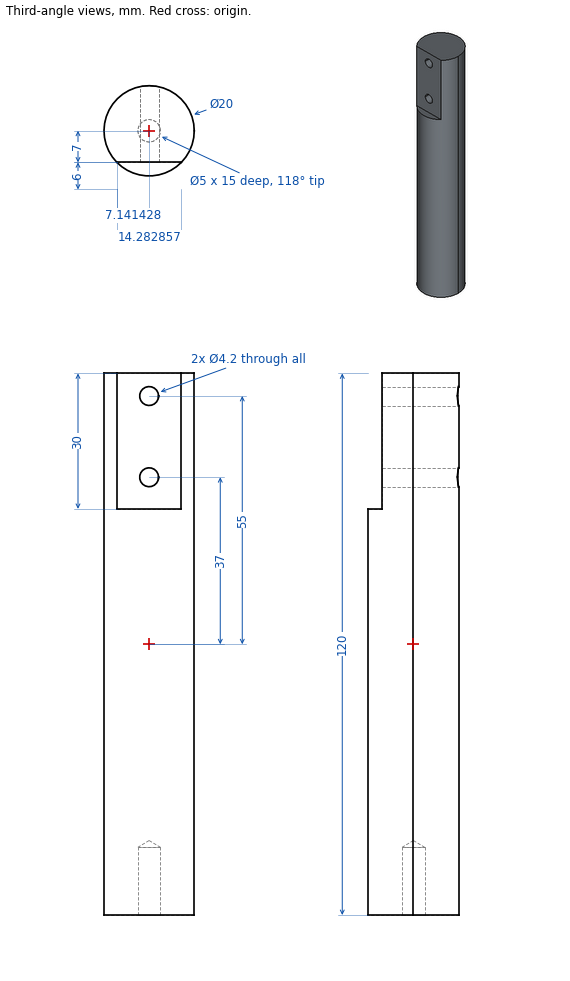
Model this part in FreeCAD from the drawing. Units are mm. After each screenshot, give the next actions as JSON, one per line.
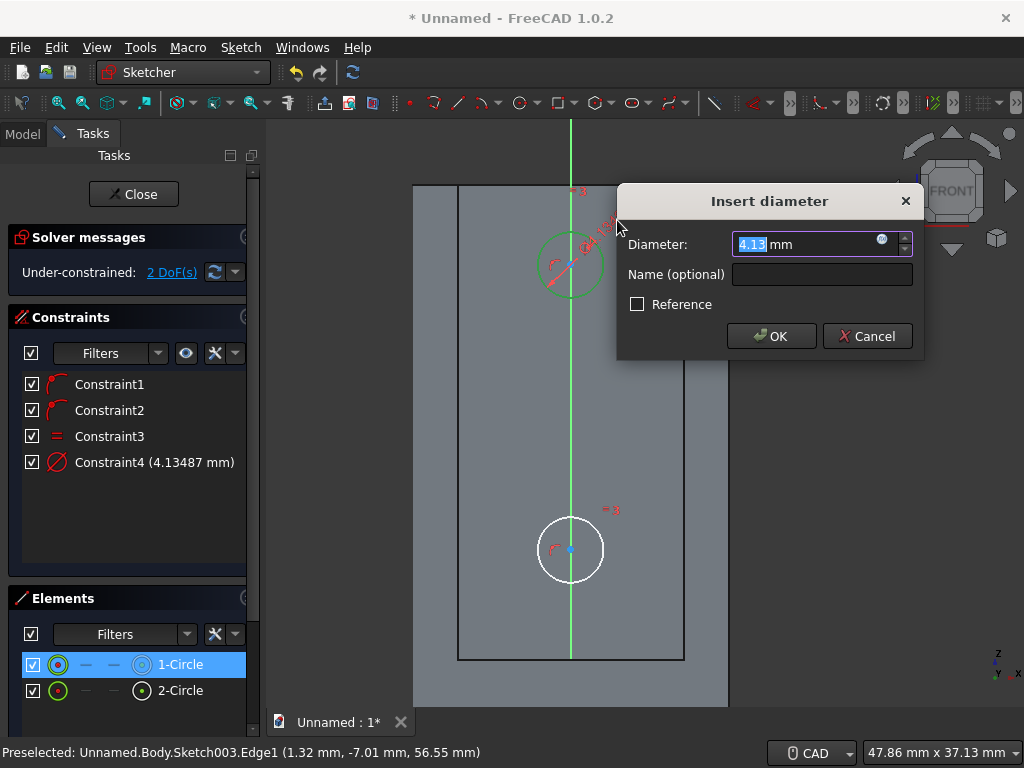
{"action": "type", "text": "4.2"}
{"action": "key", "text": "Return"}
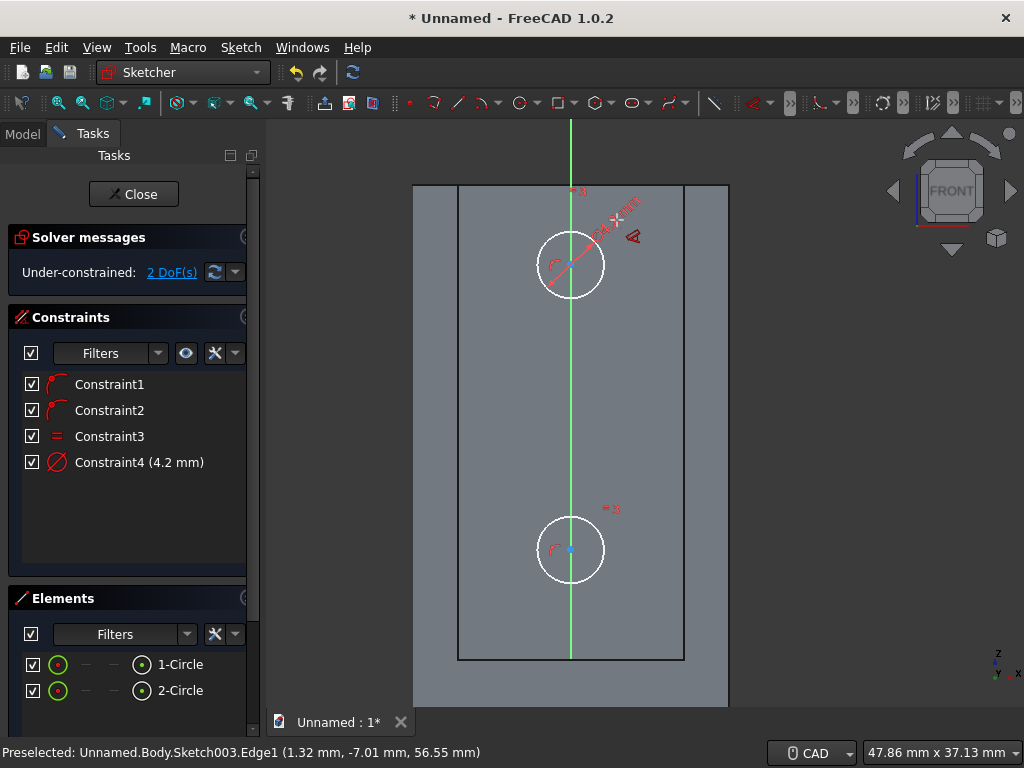
{"action": "left_click", "coordinate": [571, 265]}
{"action": "left_click", "coordinate": [605, 472]}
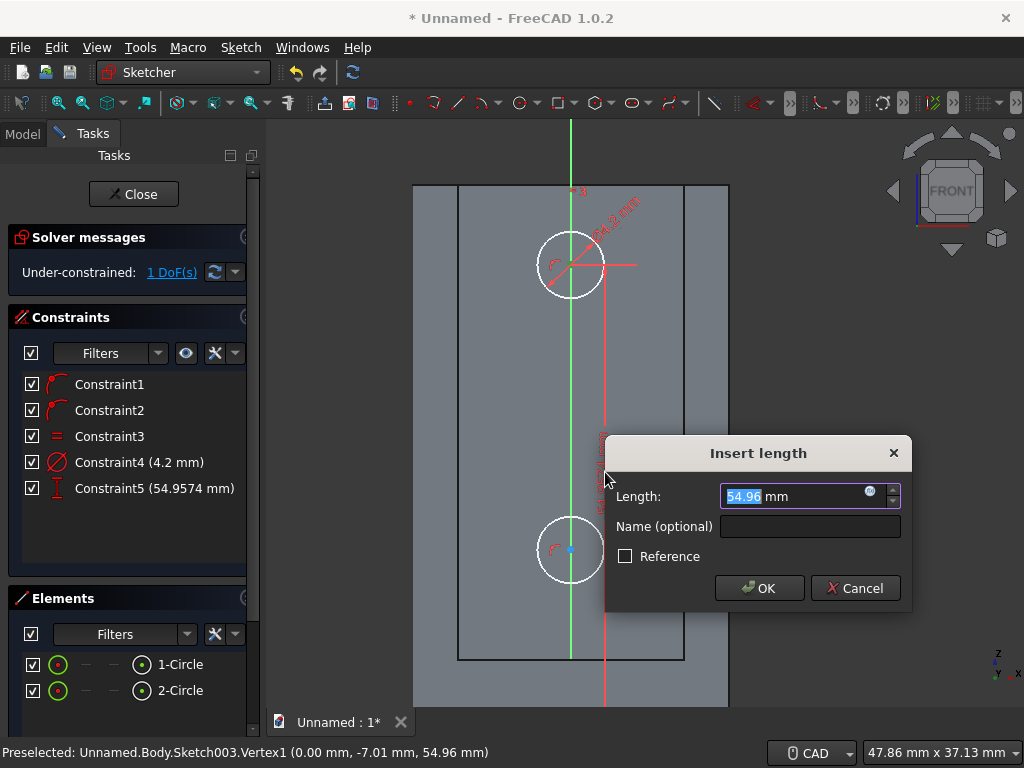
{"action": "type", "text": "55"}
{"action": "key", "text": "Return"}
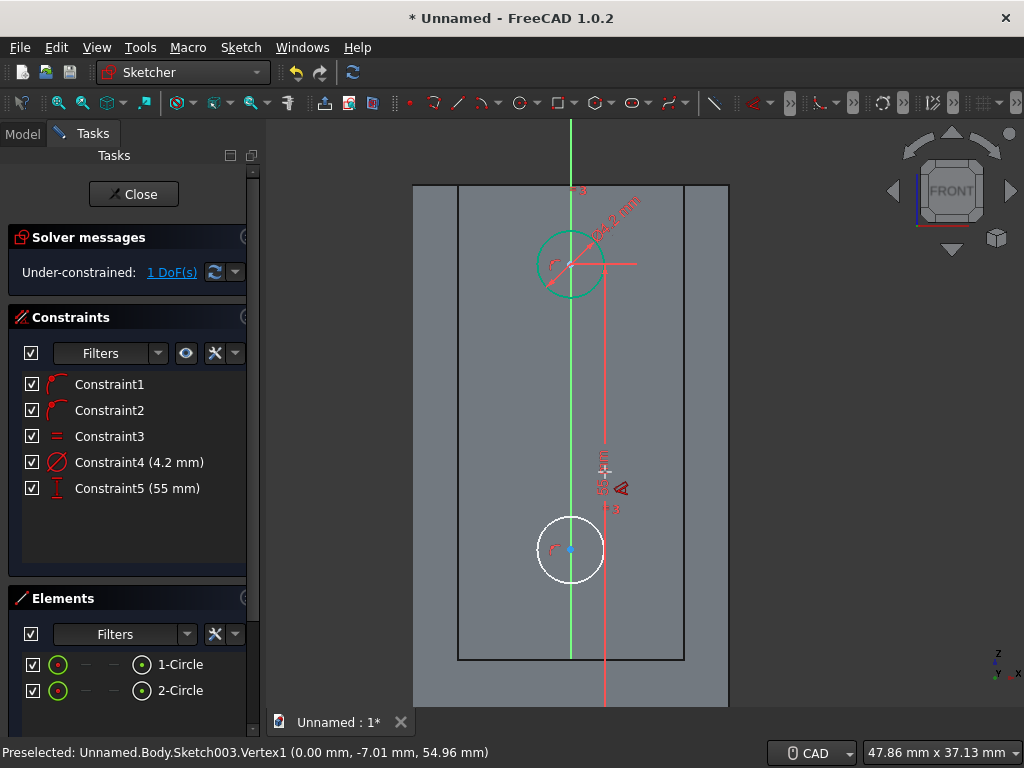
{"action": "left_click", "coordinate": [571, 550]}
{"action": "left_click", "coordinate": [605, 615]}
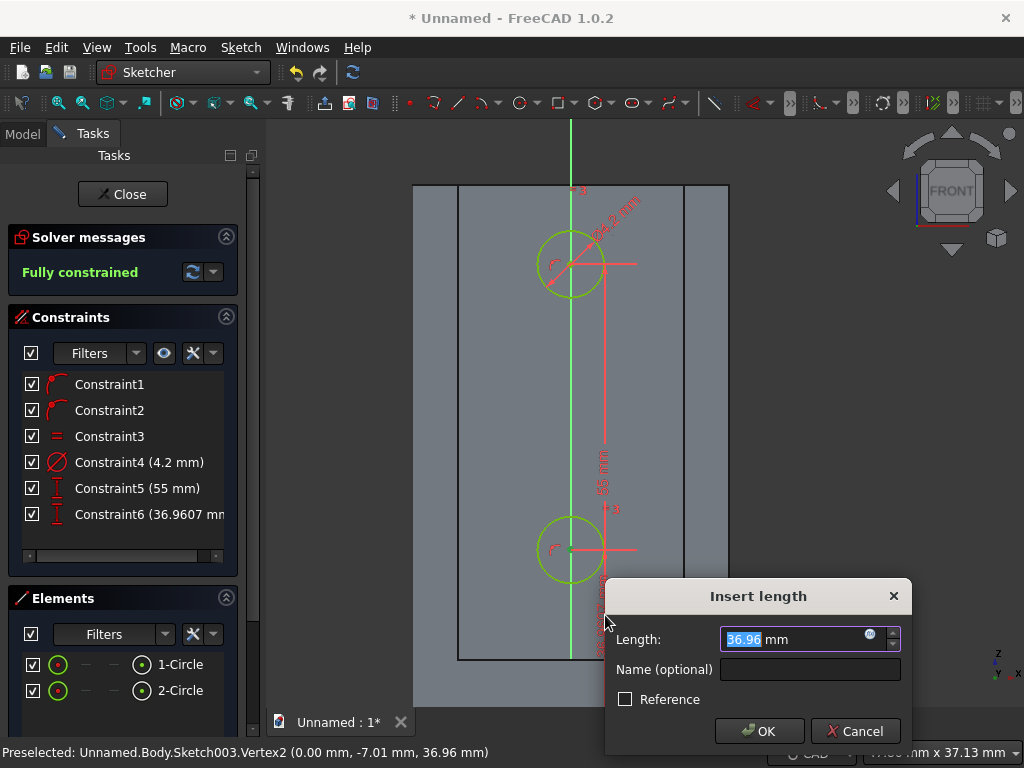
{"action": "type", "text": "37"}
{"action": "key", "text": "Return"}
{"action": "key", "text": "Escape"}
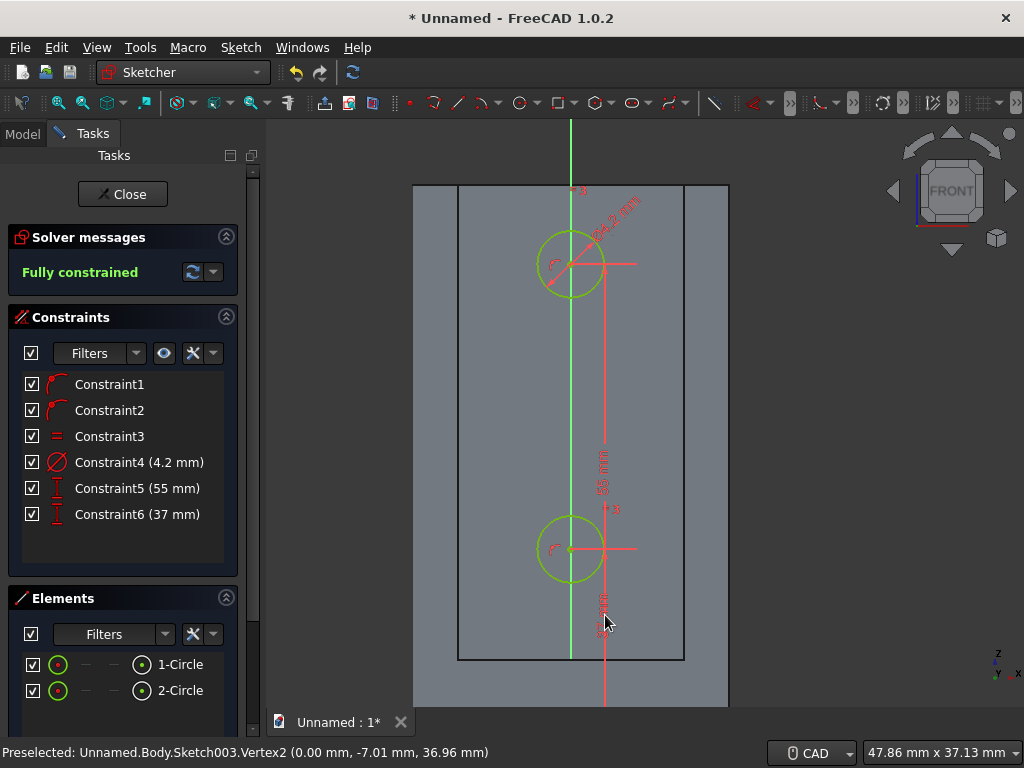
{"action": "left_click", "coordinate": [123, 194]}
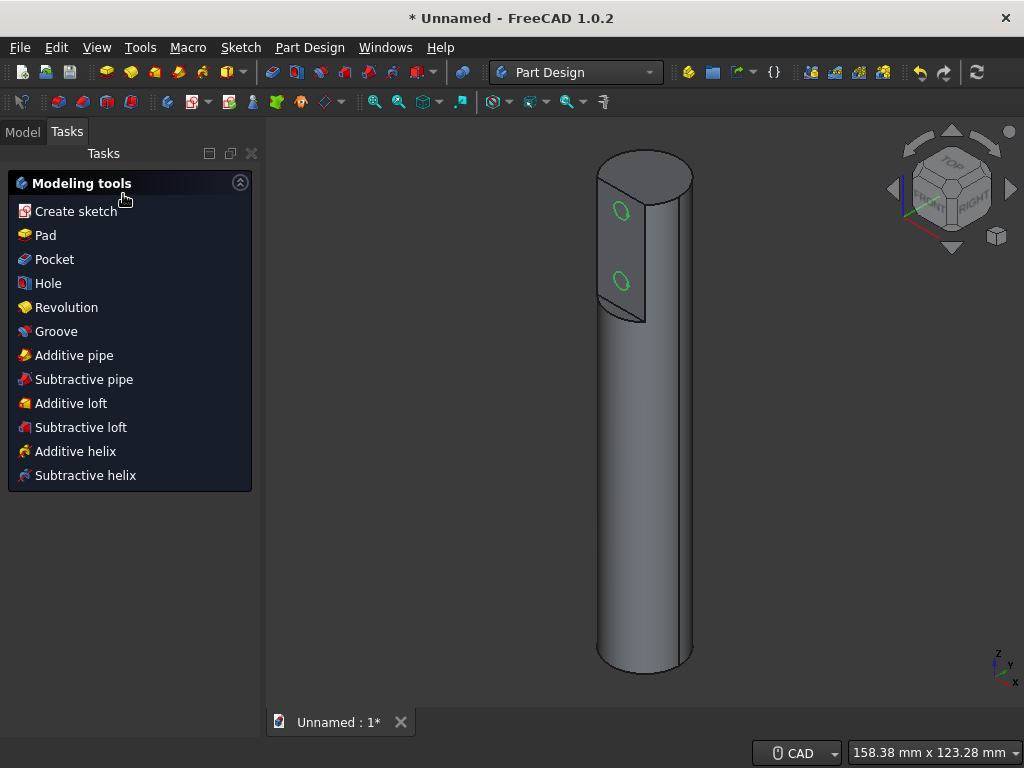
{"action": "left_click", "coordinate": [298, 72]}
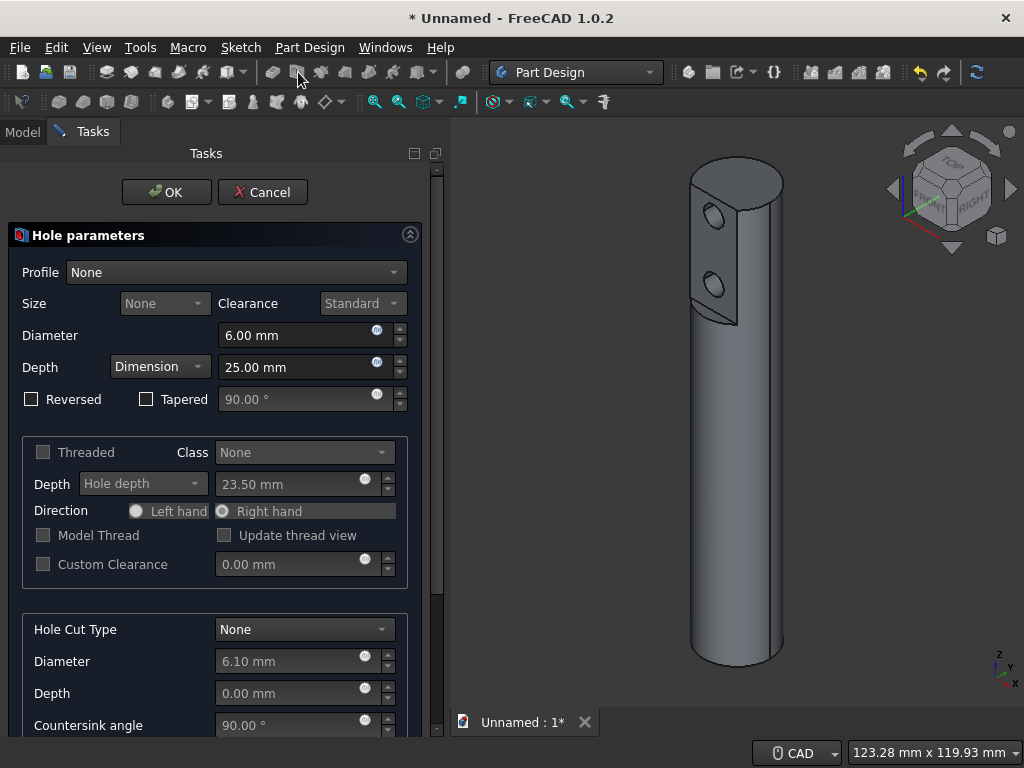
{"action": "triple_click", "coordinate": [305, 335]}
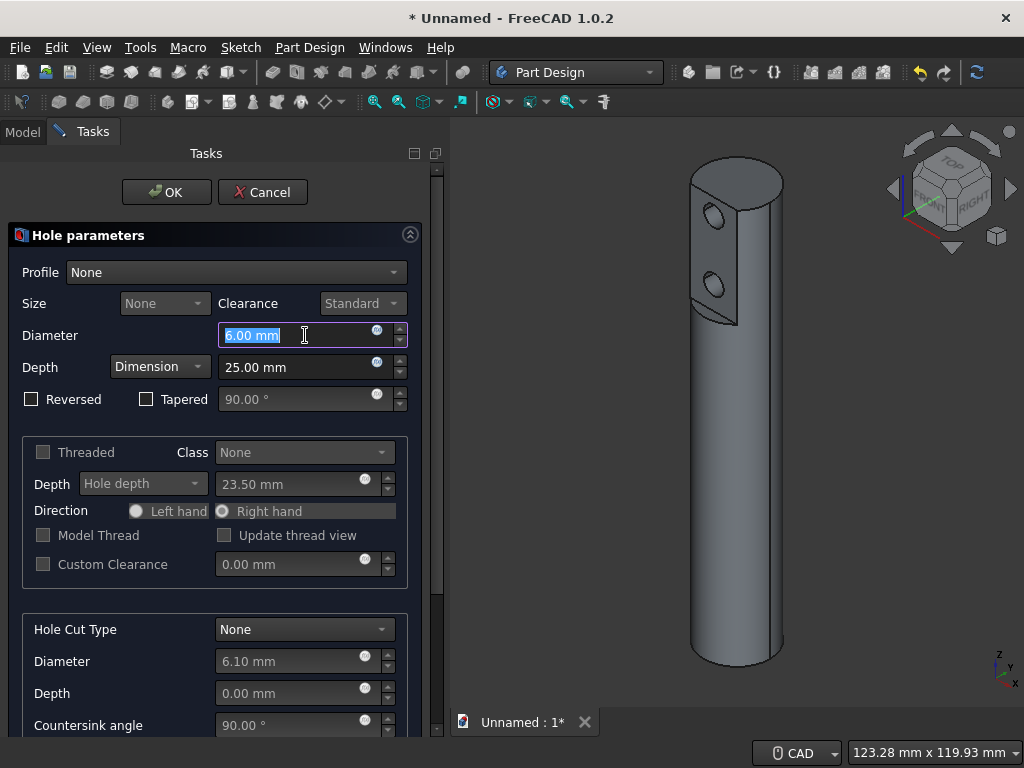
{"action": "type", "text": "4.2"}
{"action": "key", "text": "Tab"}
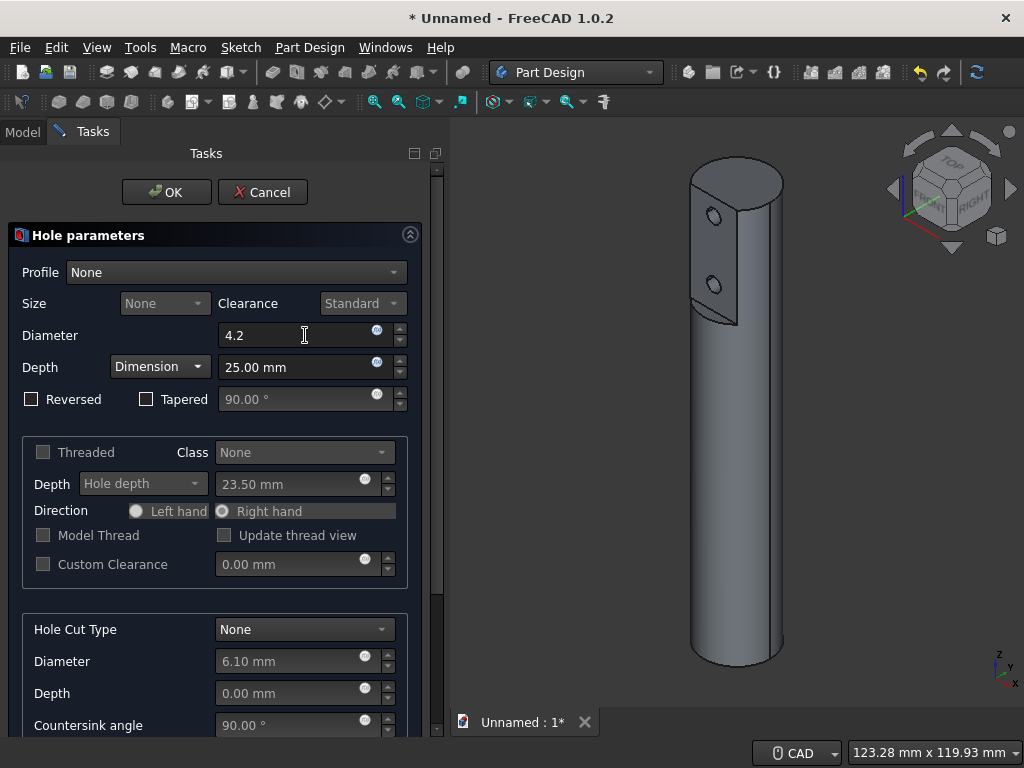
{"action": "left_click", "coordinate": [161, 366]}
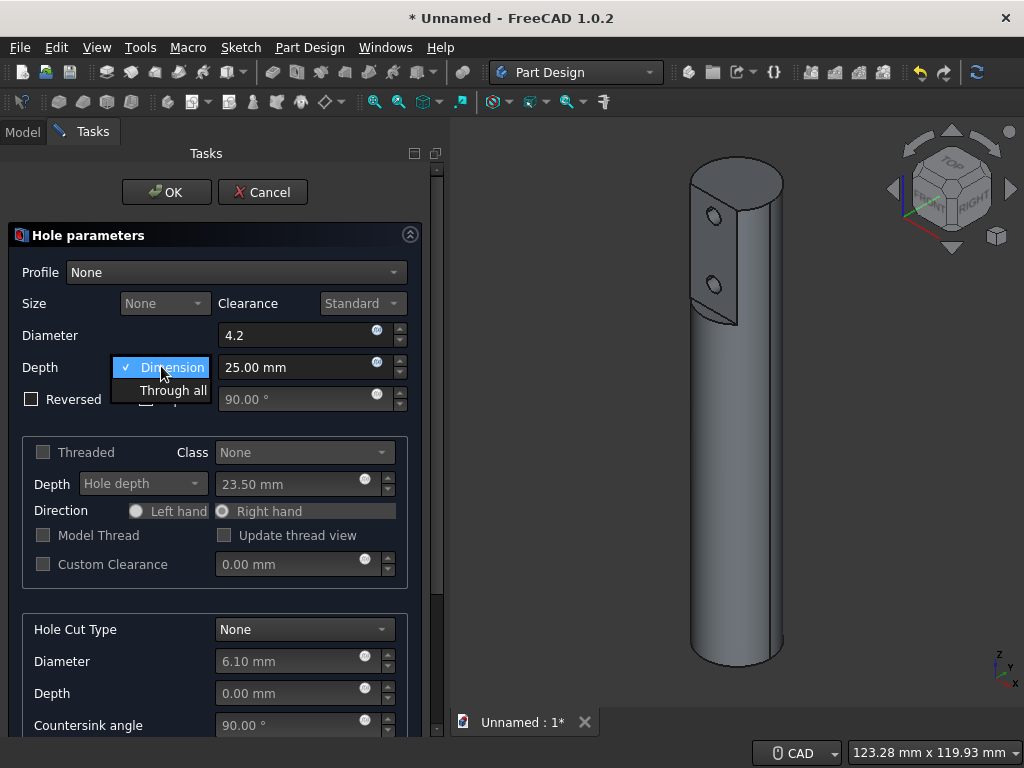
{"action": "left_click", "coordinate": [160, 390]}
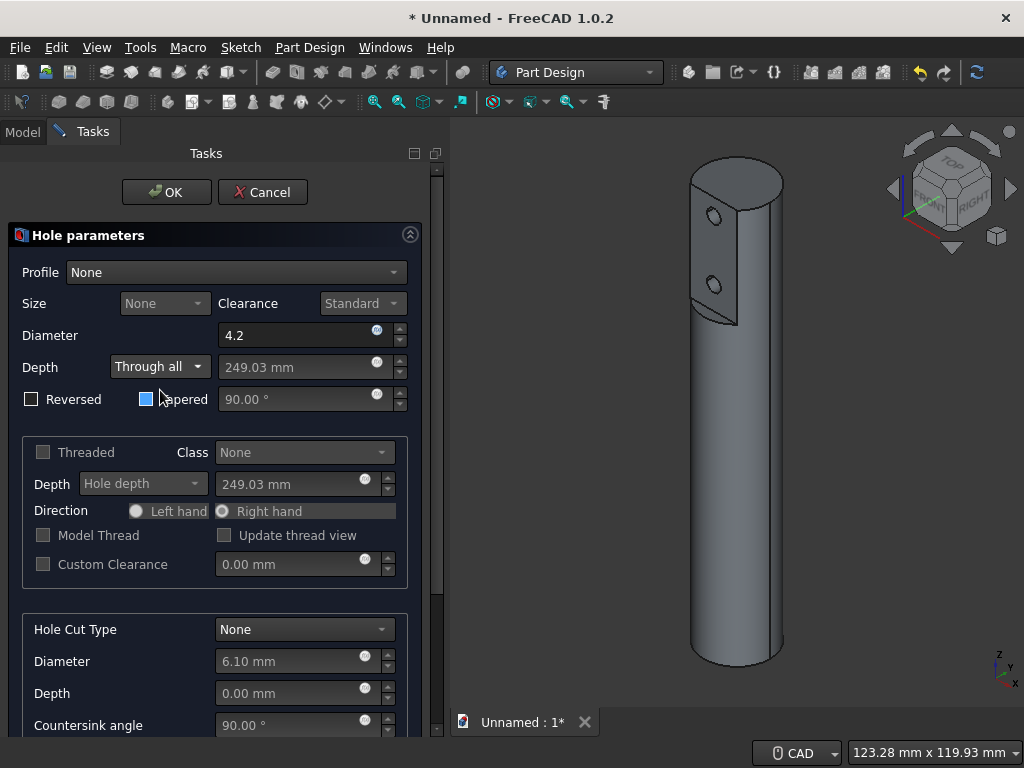
{"action": "left_click", "coordinate": [167, 192]}